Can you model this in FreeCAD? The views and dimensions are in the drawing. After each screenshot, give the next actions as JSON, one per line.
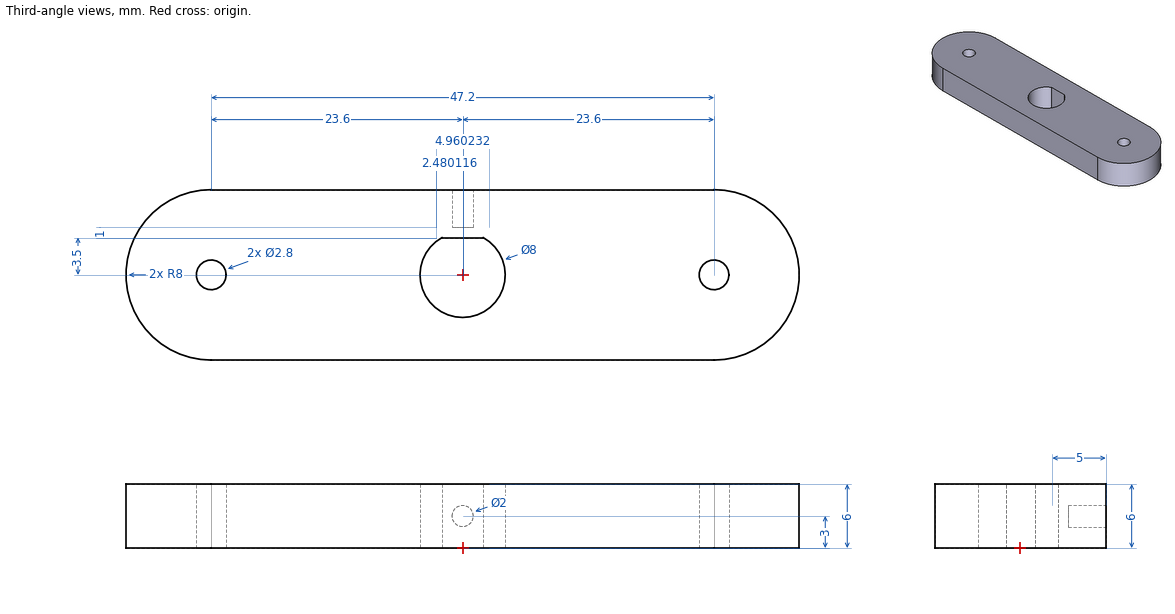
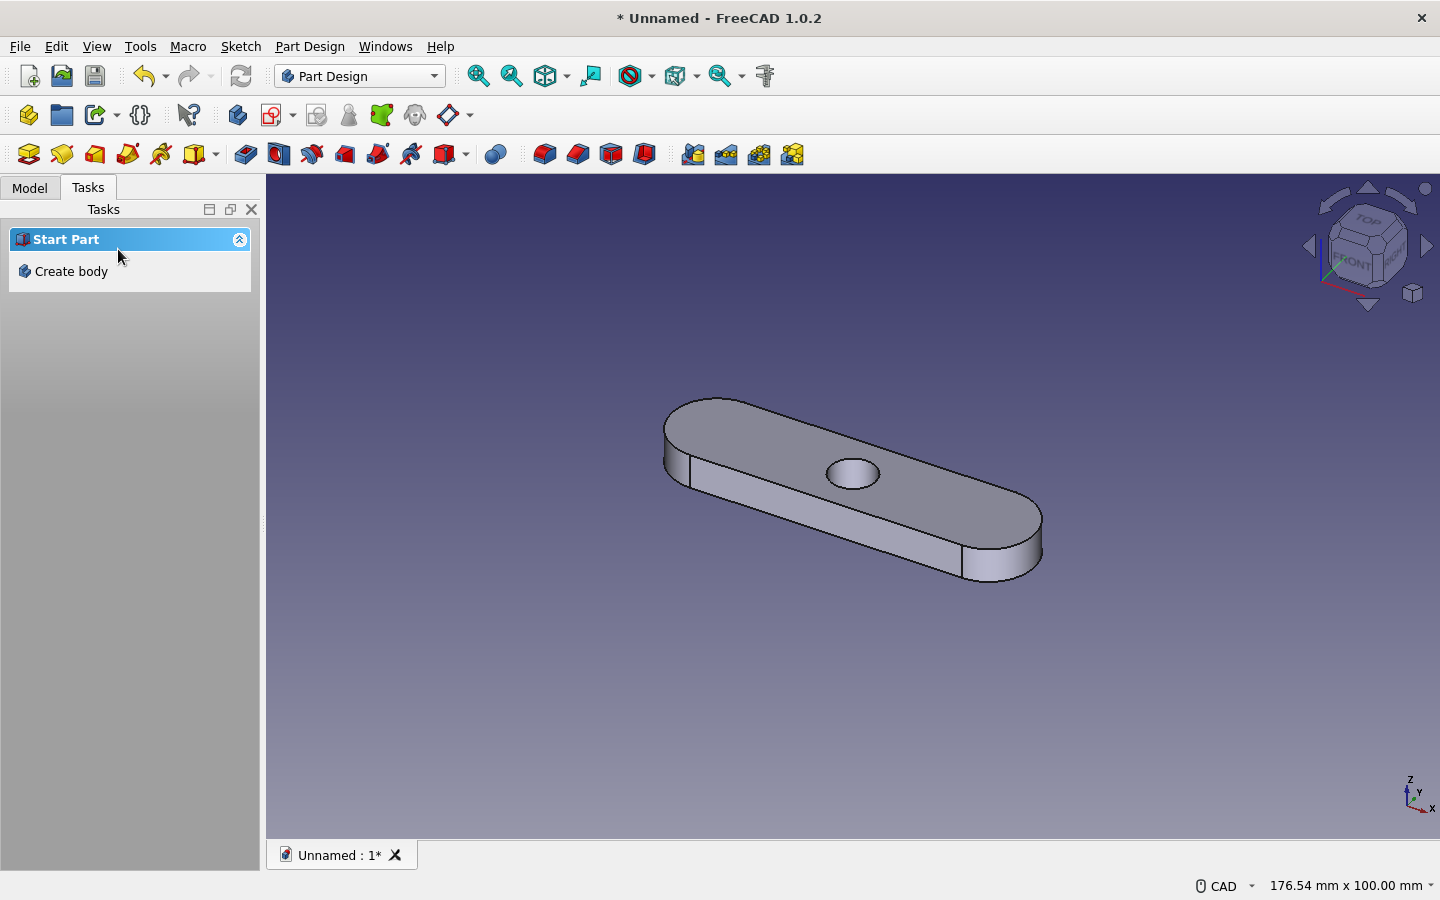
{"action": "left_click", "coordinate": [479, 76]}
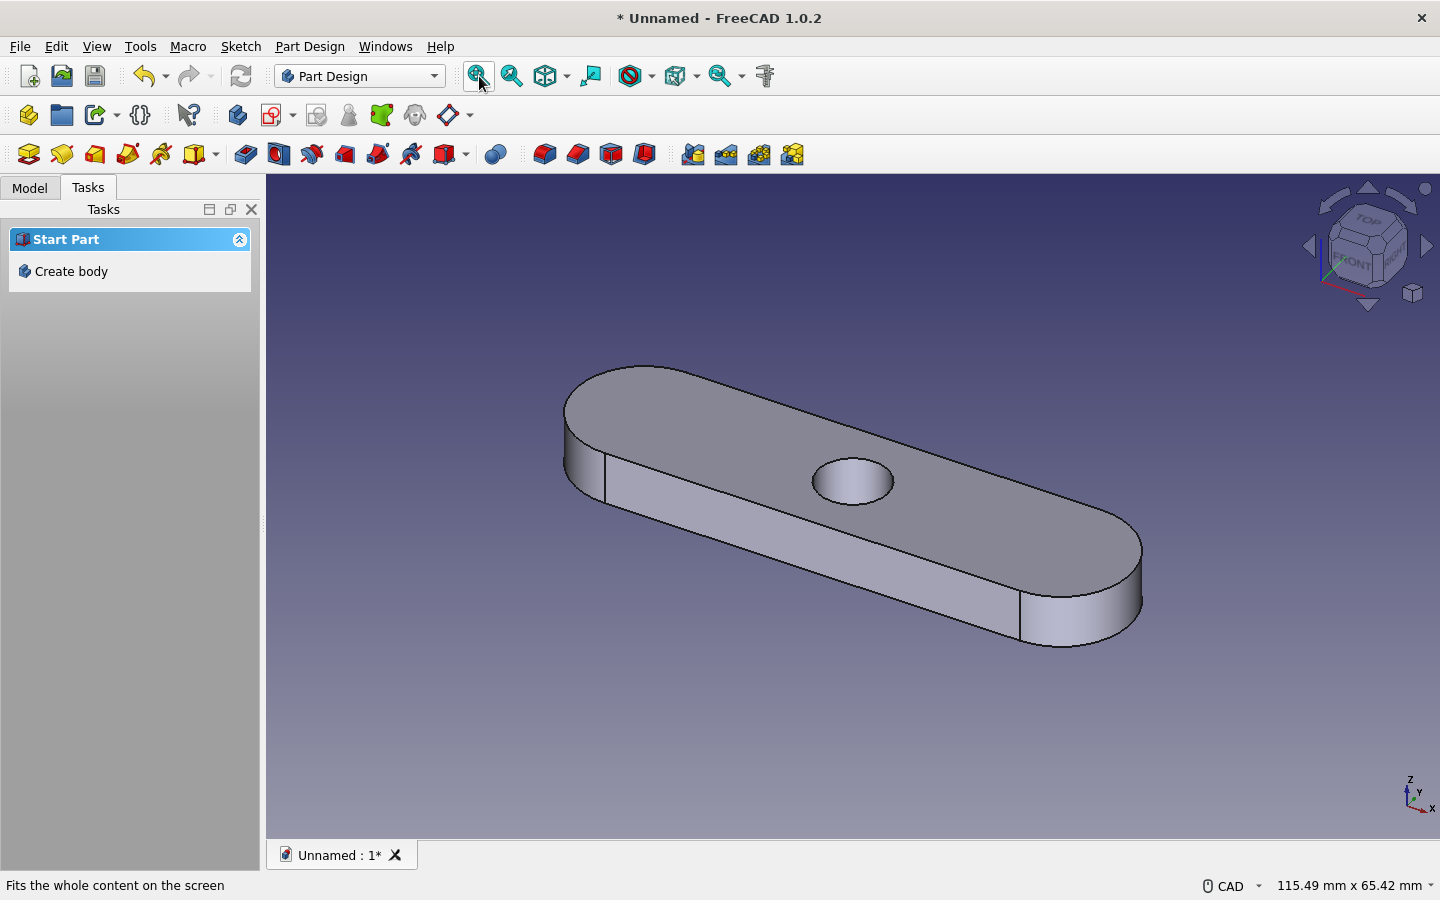
{"action": "left_click", "coordinate": [1012, 533]}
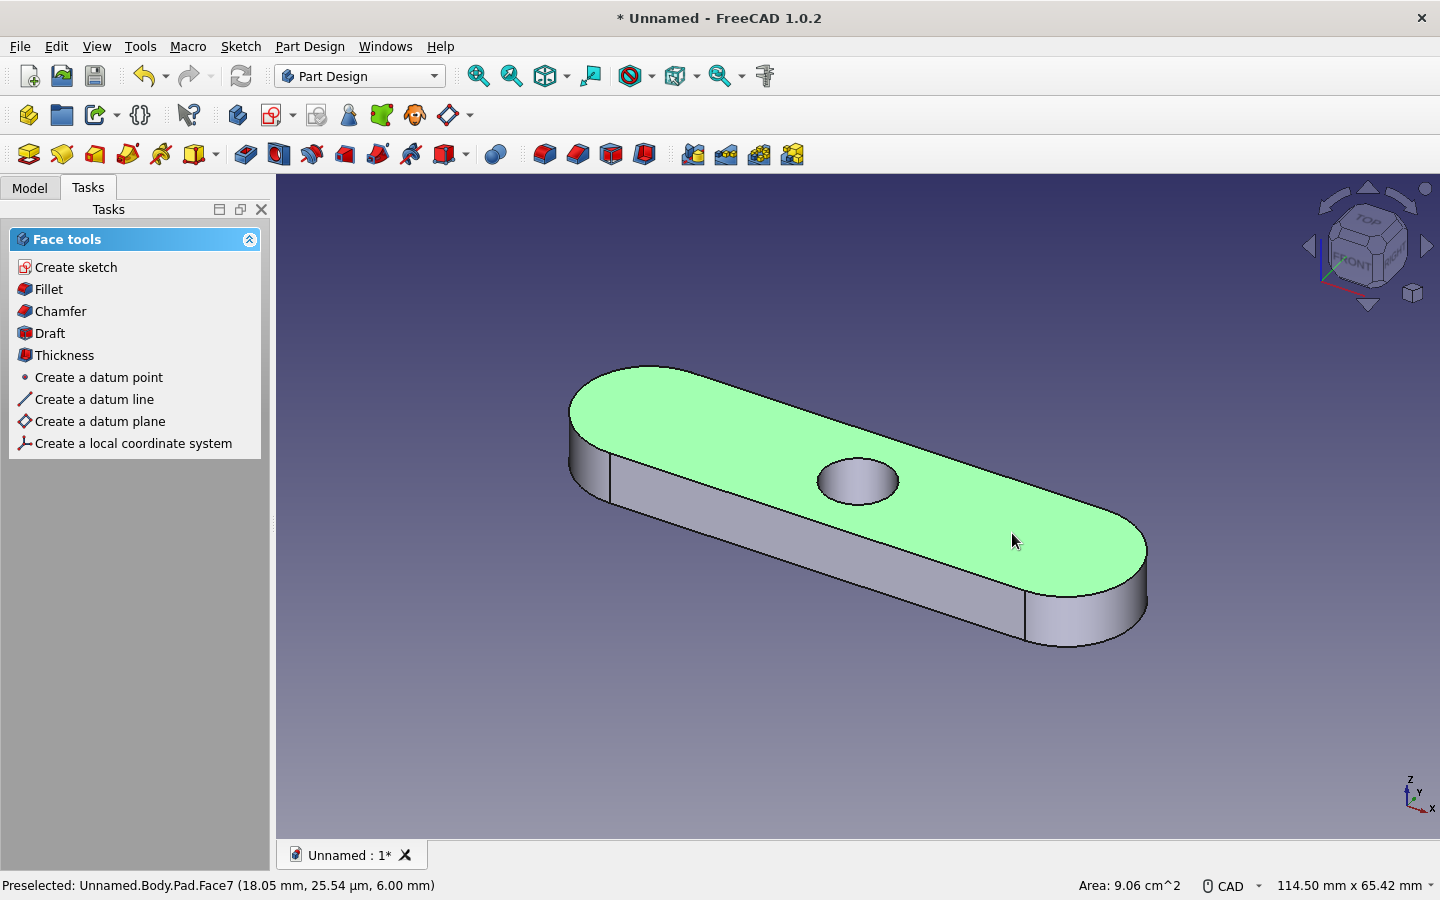
{"action": "left_click", "coordinate": [270, 116]}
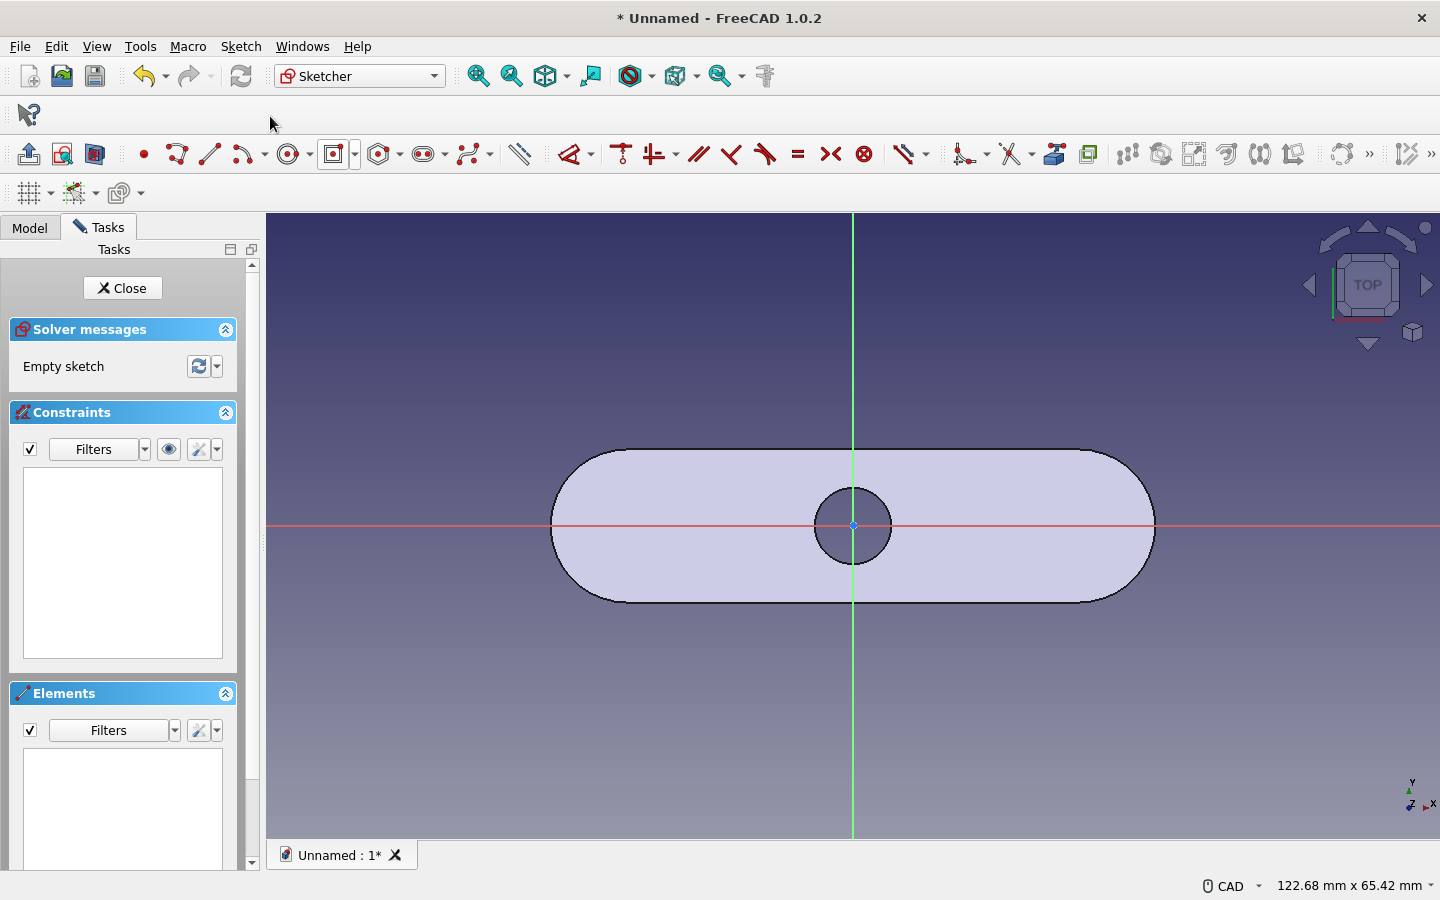
{"action": "scroll", "coordinate": [992, 526], "scroll_direction": "up", "scroll_amount": 2}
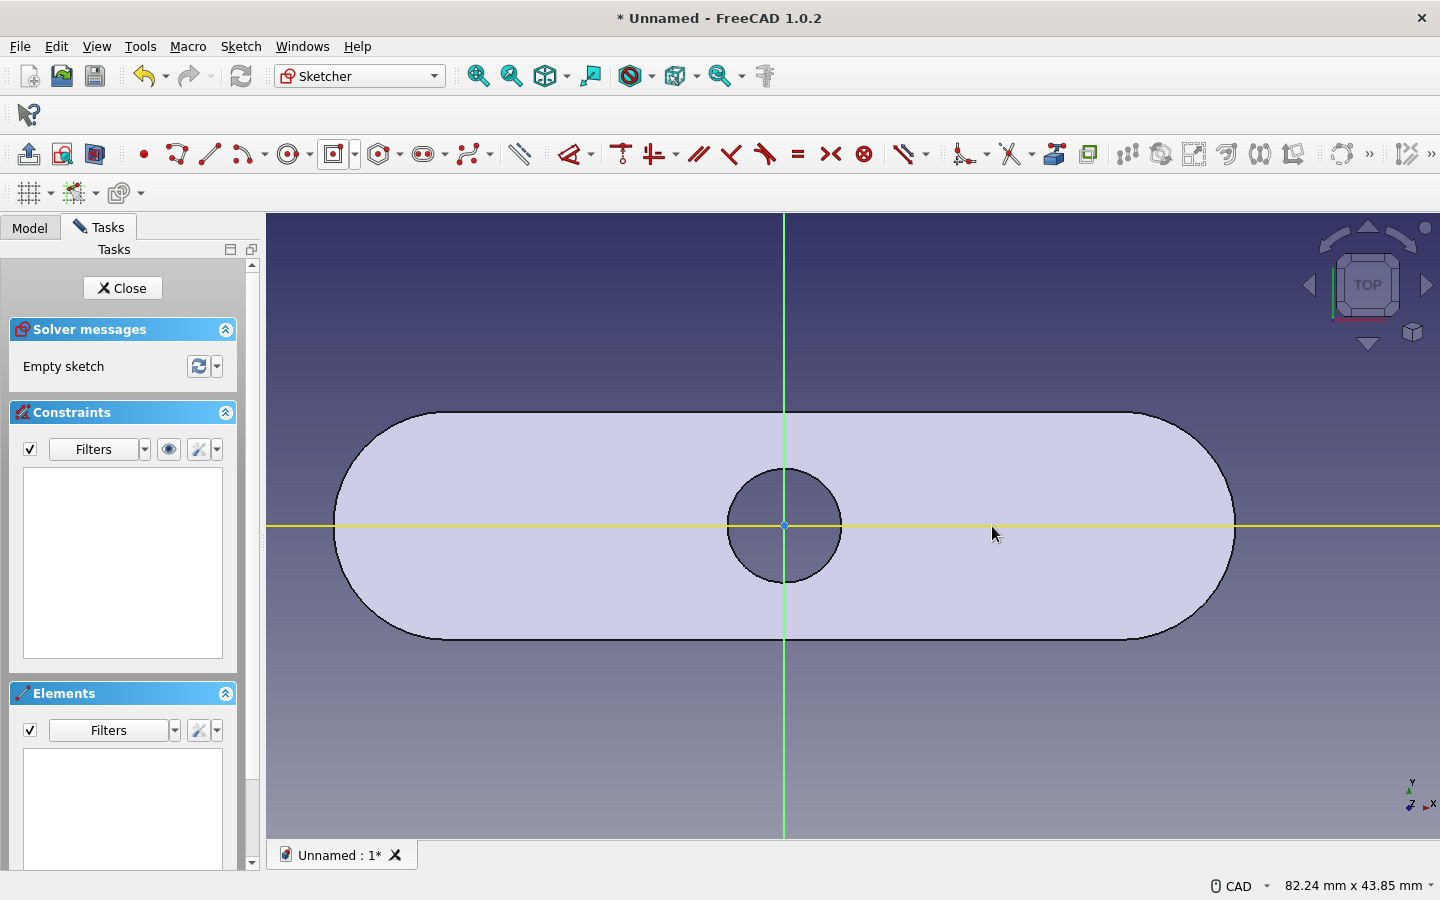
{"action": "left_click", "coordinate": [288, 154]}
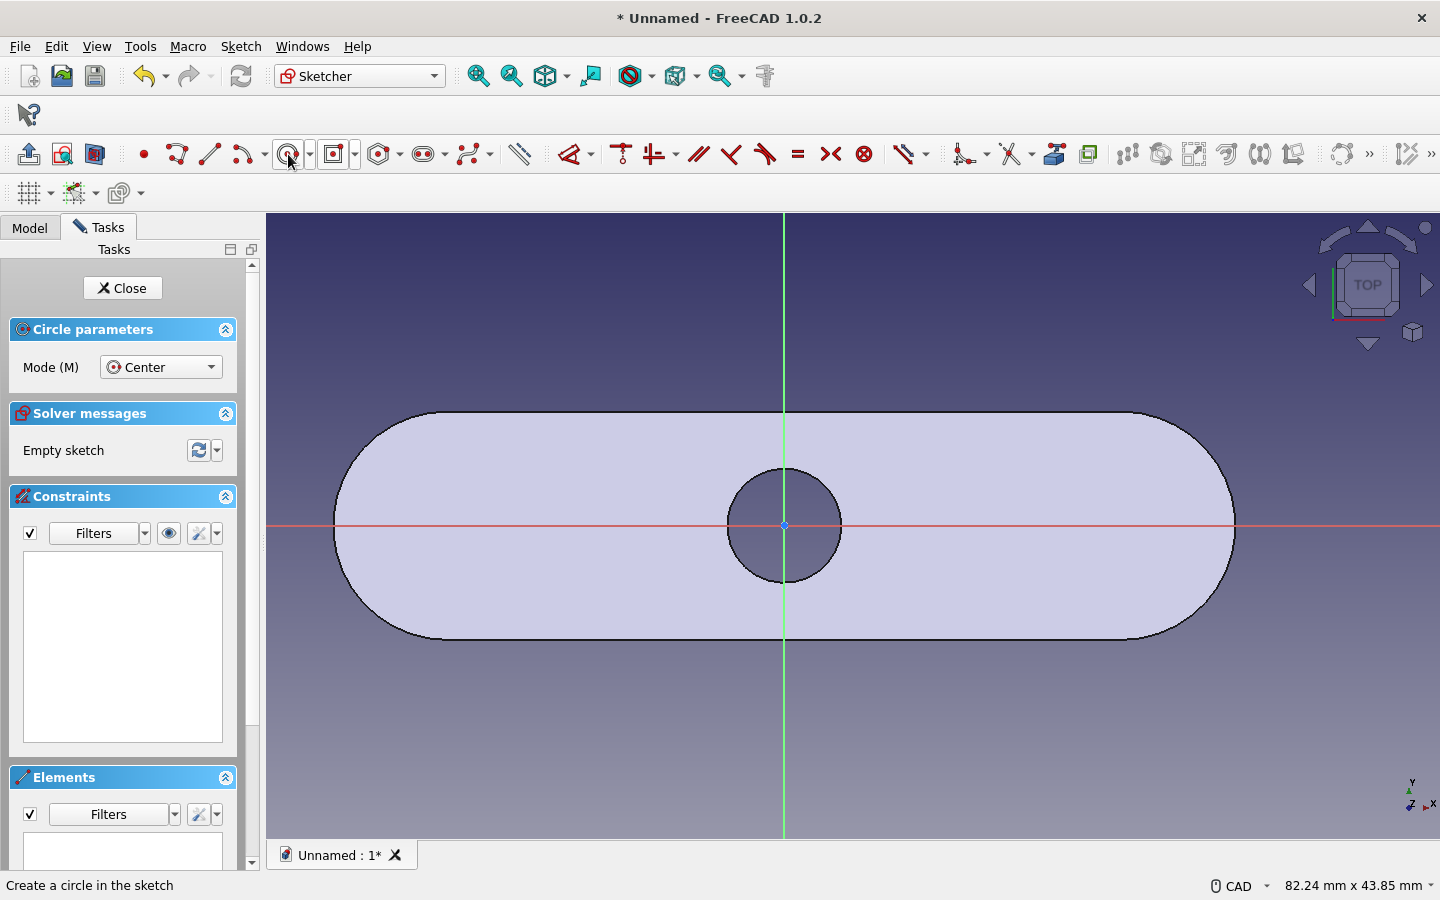
{"action": "left_click", "coordinate": [447, 526]}
{"action": "left_click", "coordinate": [462, 512]}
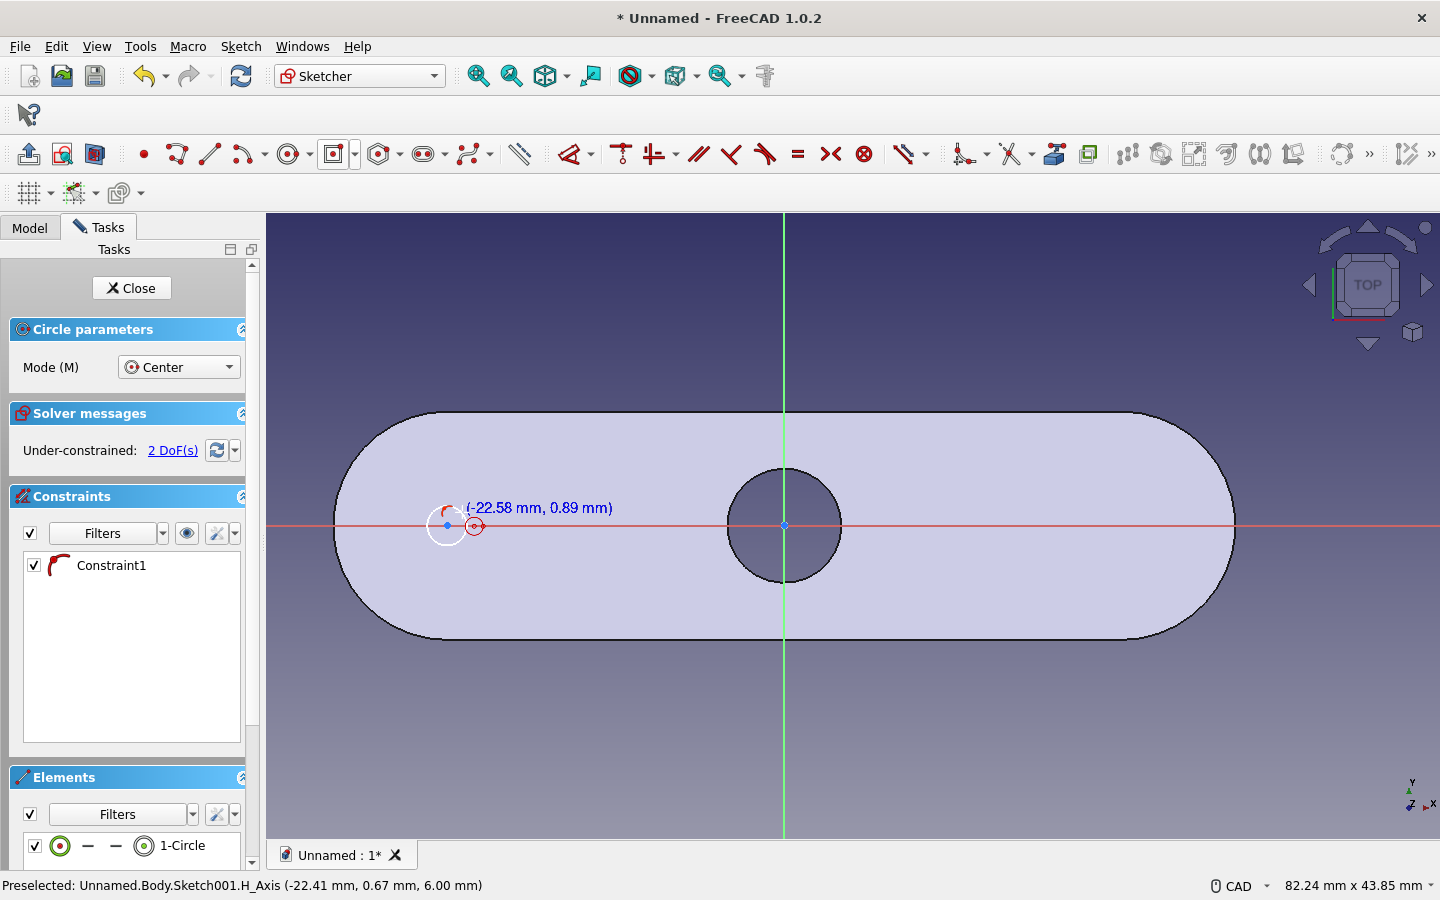
{"action": "left_click", "coordinate": [1121, 526]}
{"action": "left_click", "coordinate": [1135, 512]}
{"action": "key", "text": "Escape"}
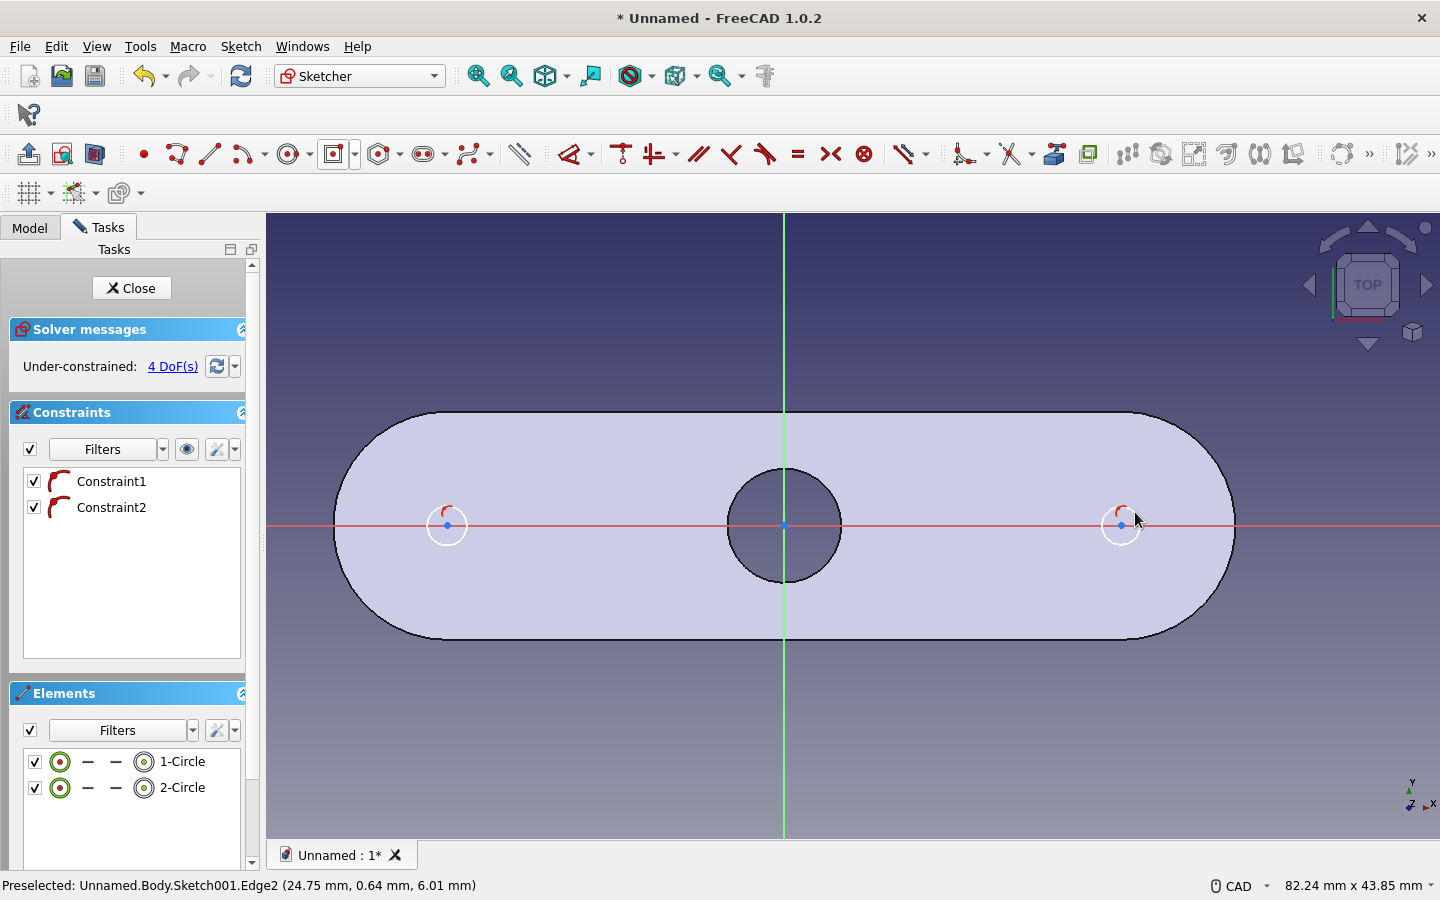
{"action": "left_click", "coordinate": [461, 512]}